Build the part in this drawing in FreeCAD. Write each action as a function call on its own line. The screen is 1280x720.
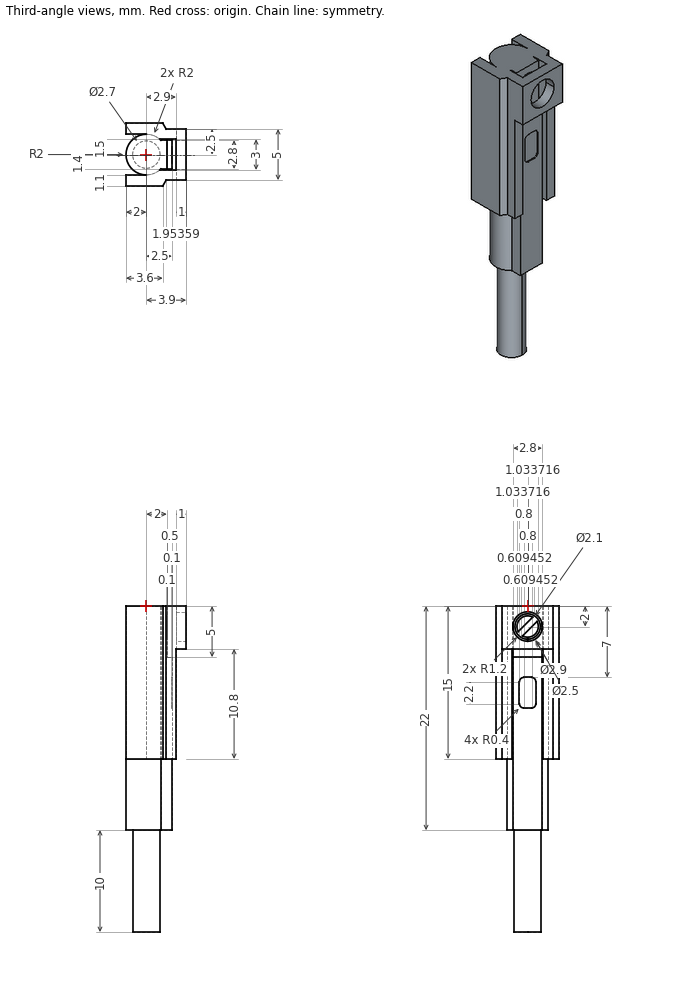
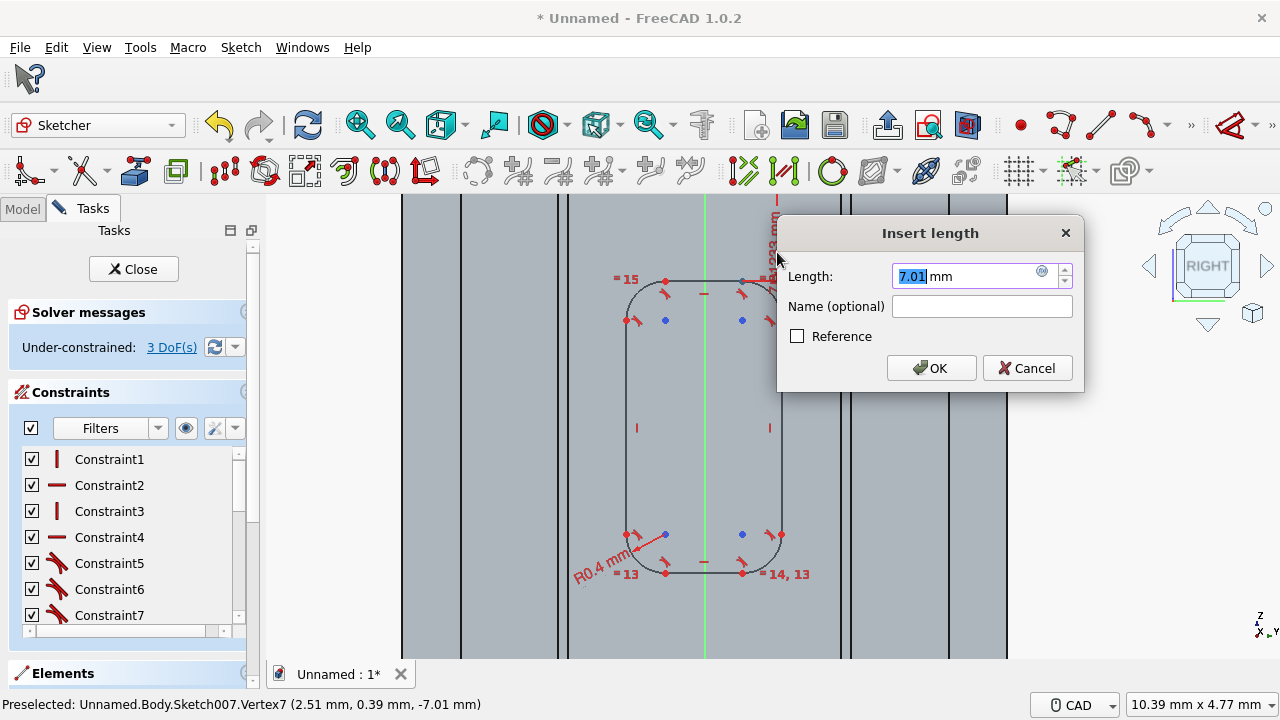
text(7)
key(Return)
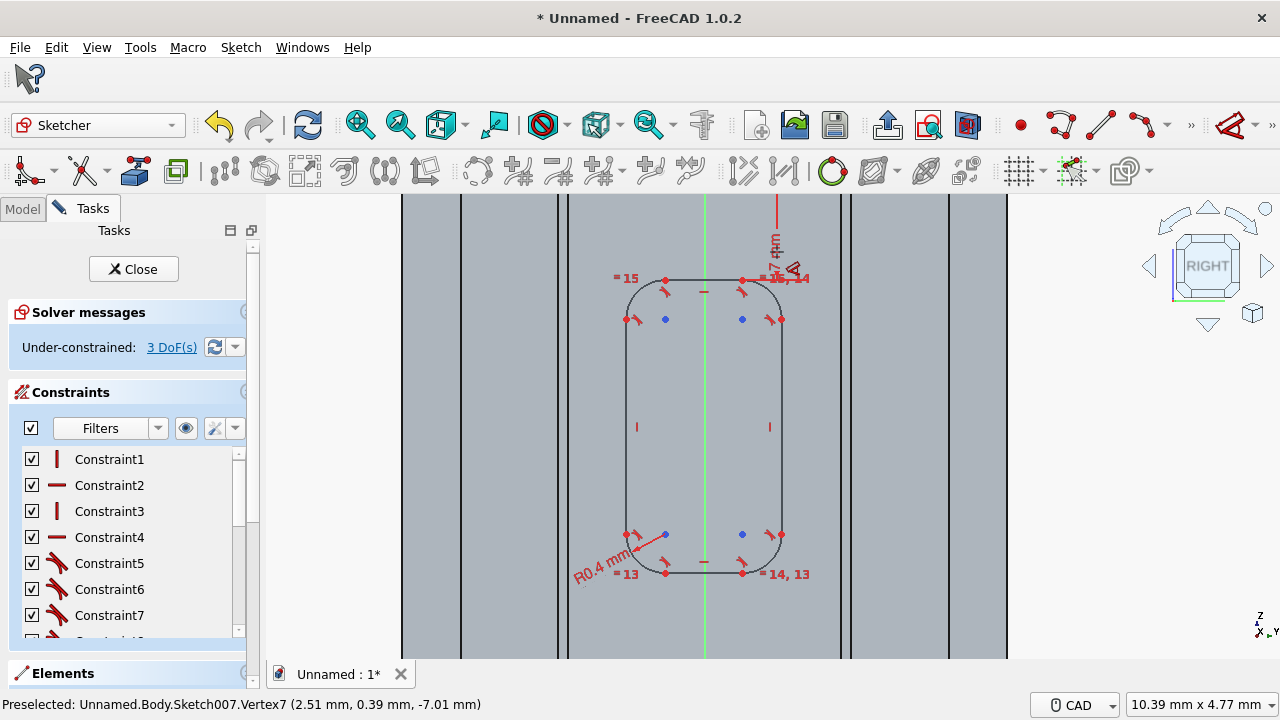
click(626, 384)
click(592, 427)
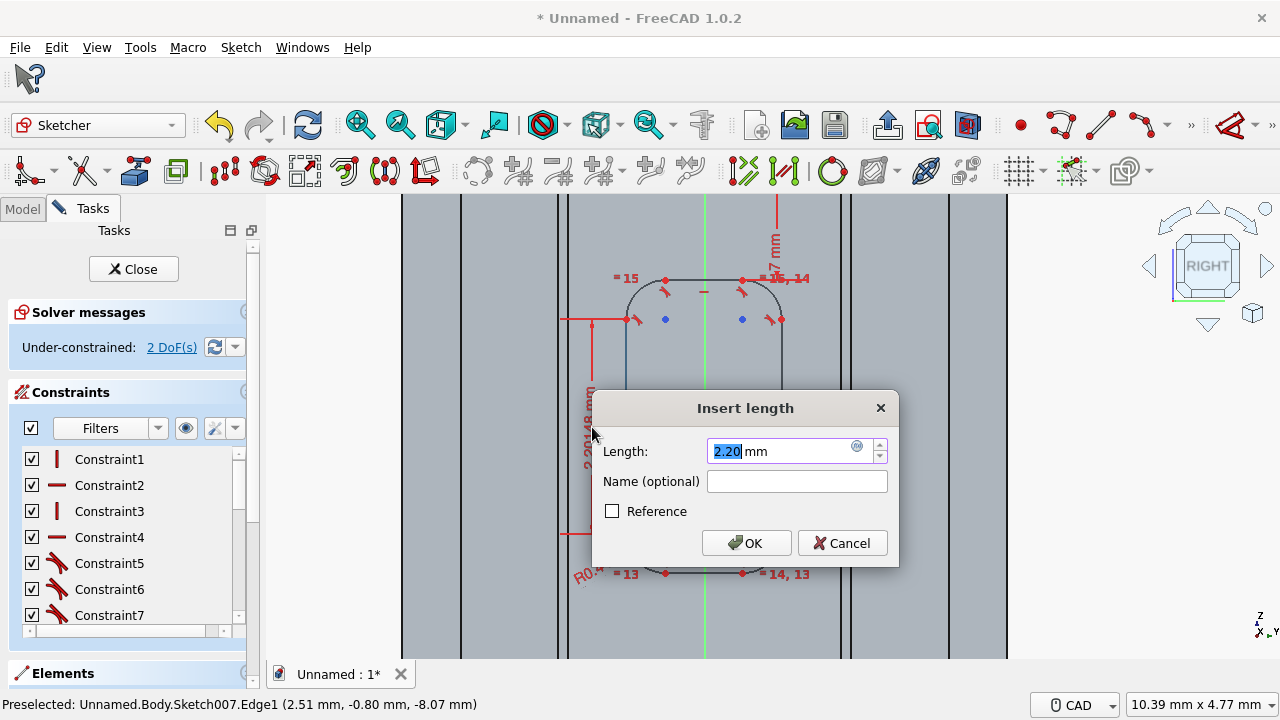
text(2.2)
key(Return)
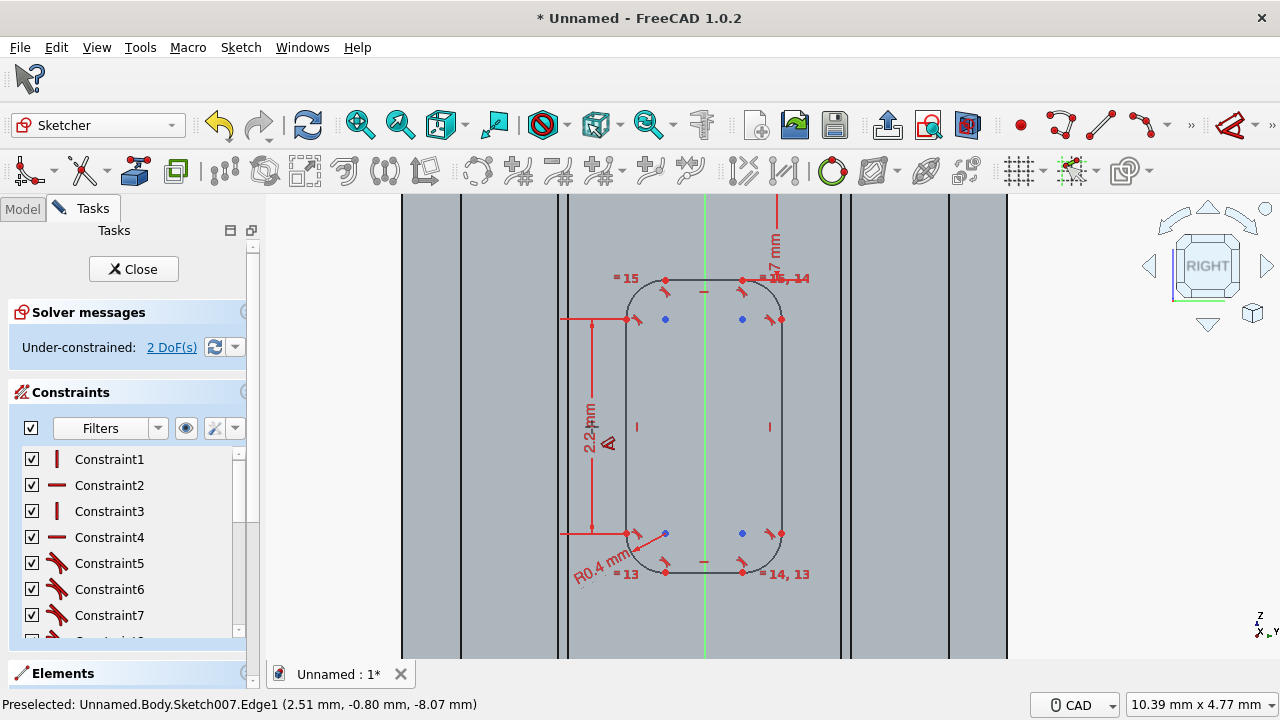
click(689, 573)
click(686, 607)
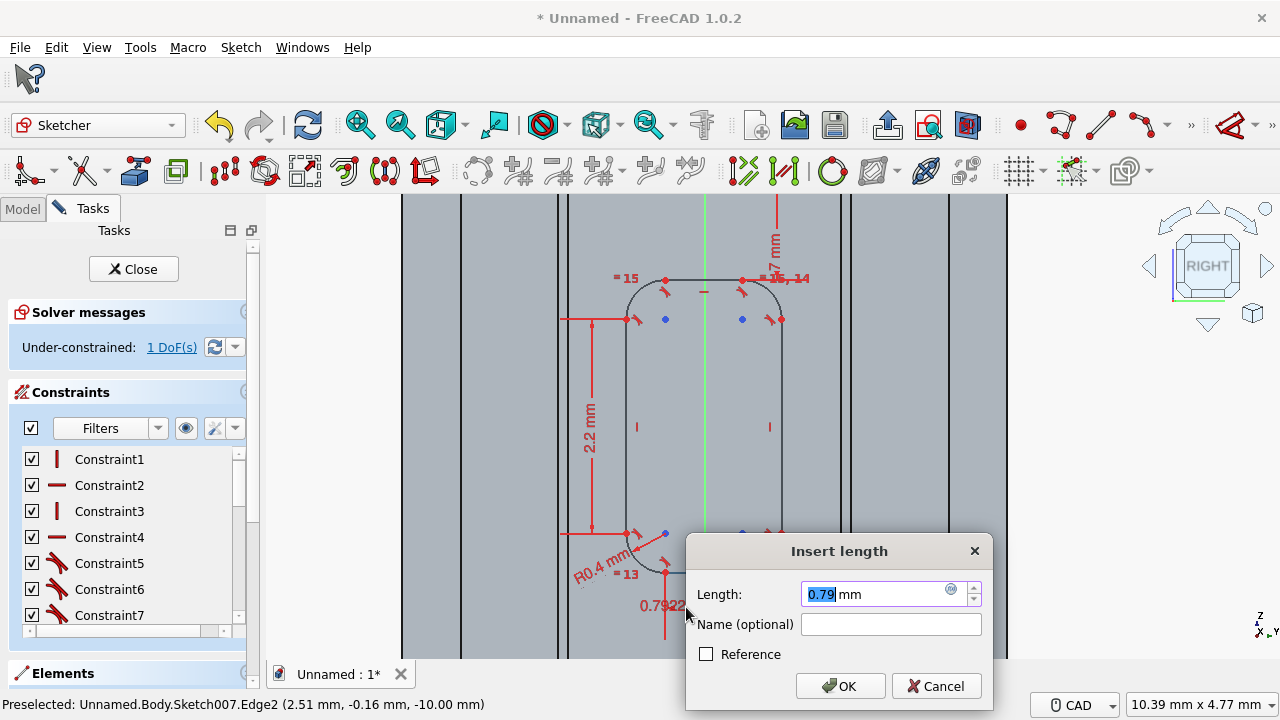
text(0.8)
key(Return)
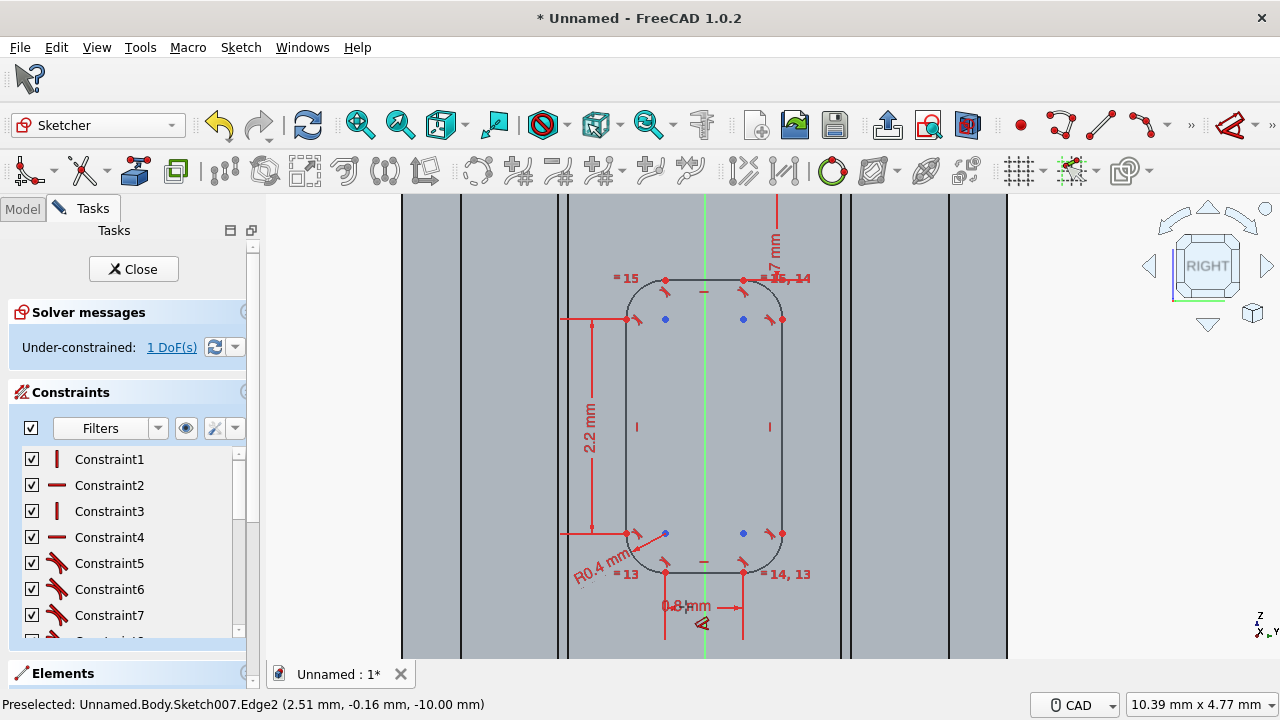
click(626, 319)
click(666, 353)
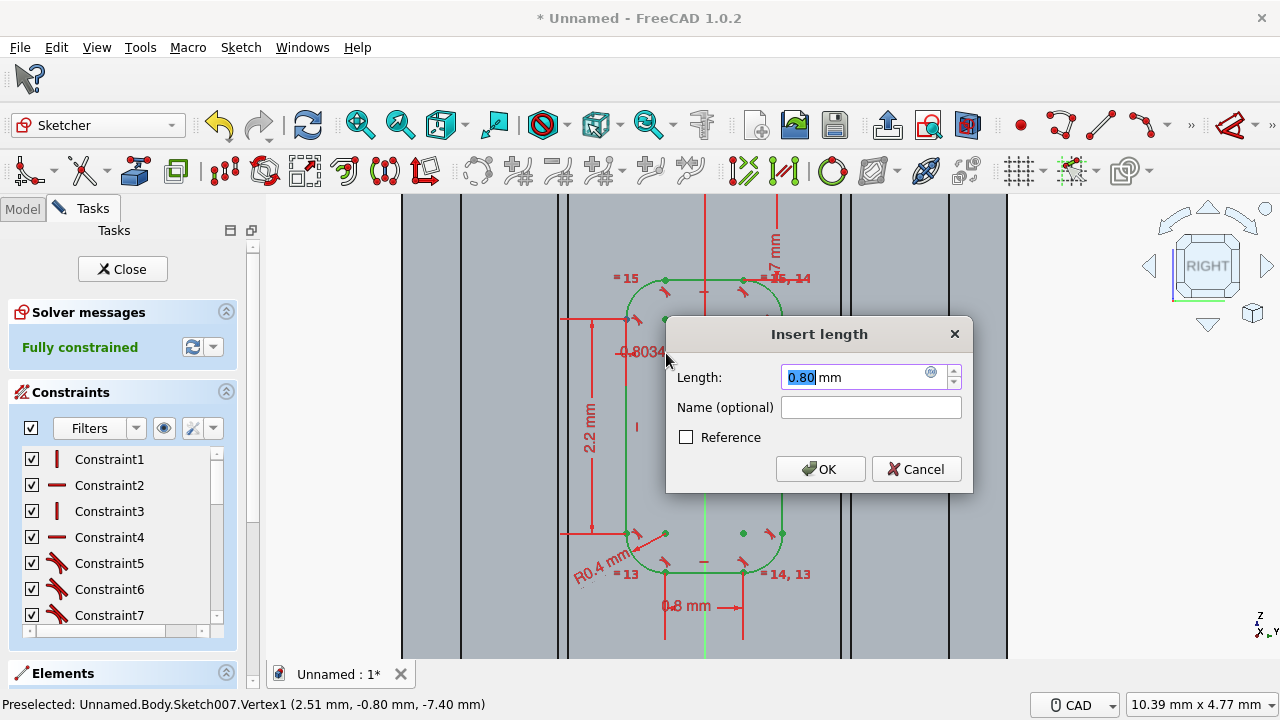
text(0.8)
key(Return)
key(Escape)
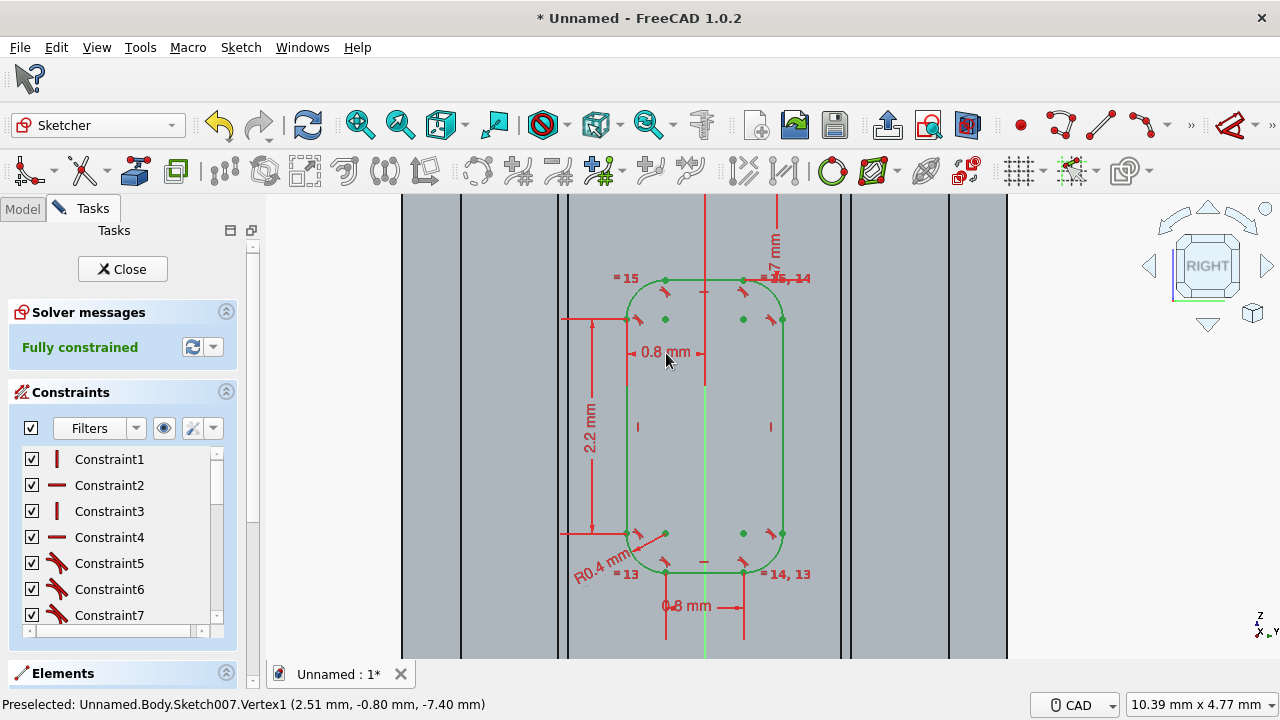
click(123, 269)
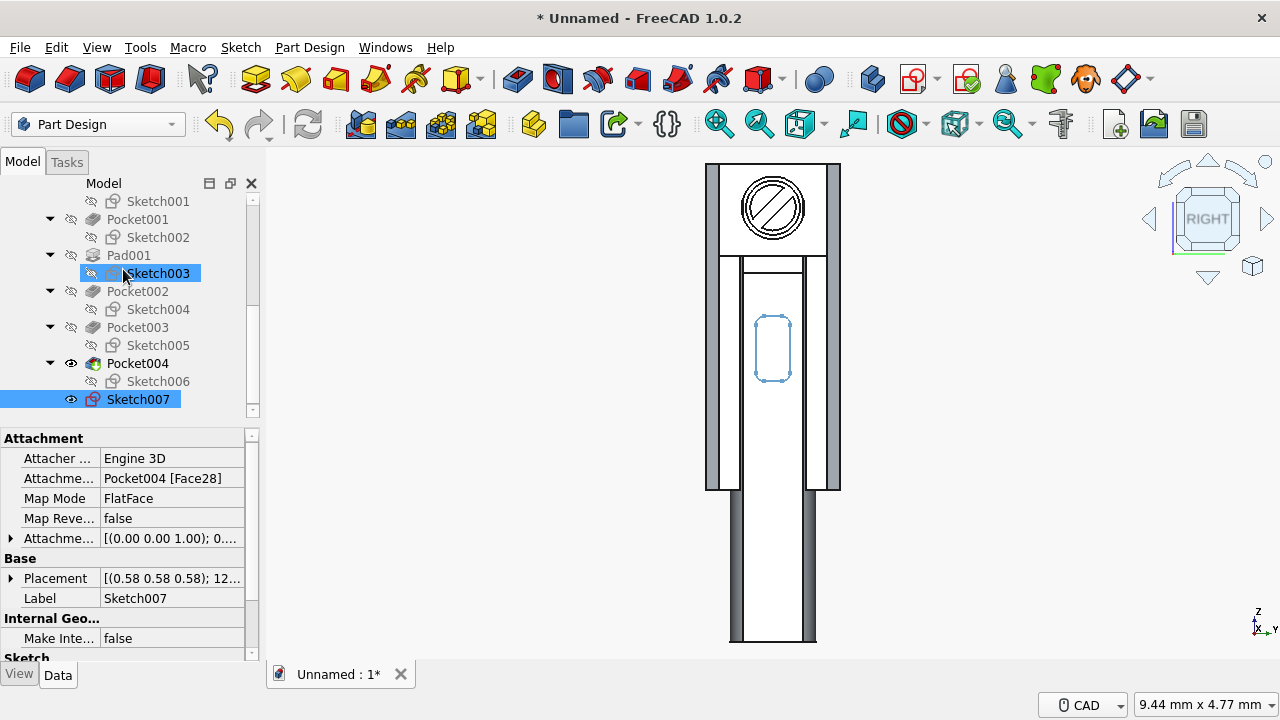
click(518, 80)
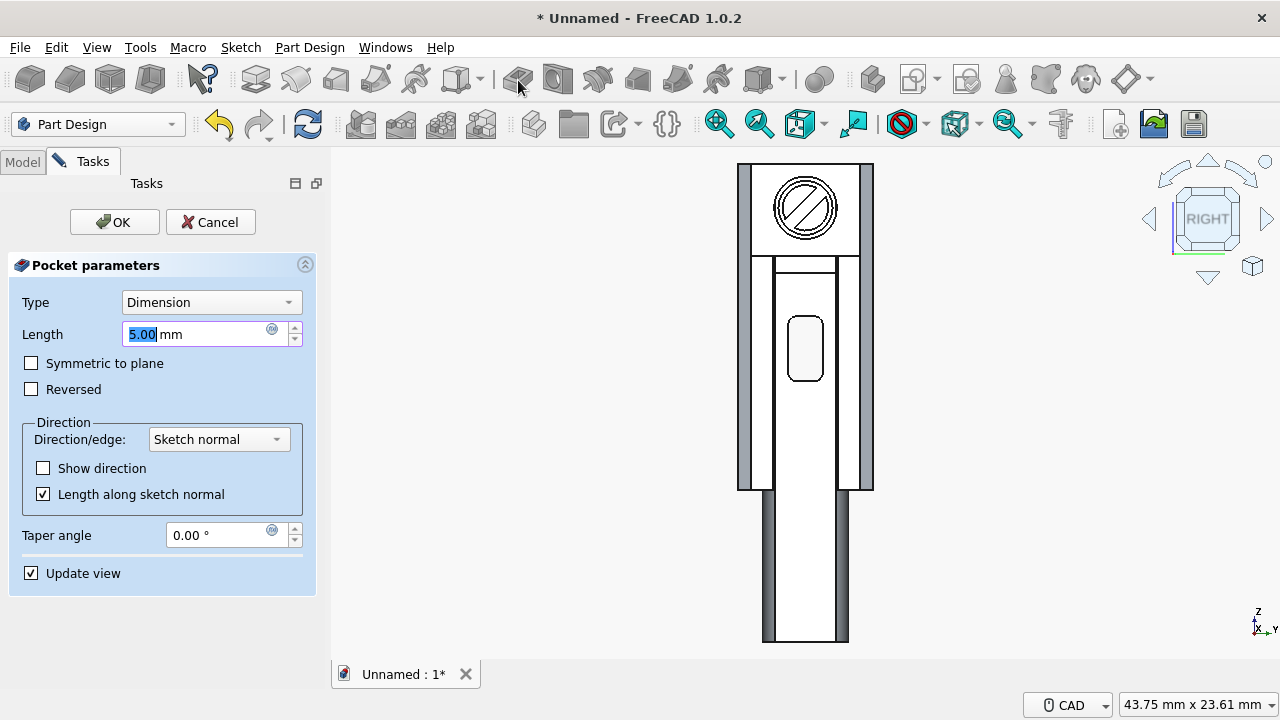
text(0.1)
key(Tab)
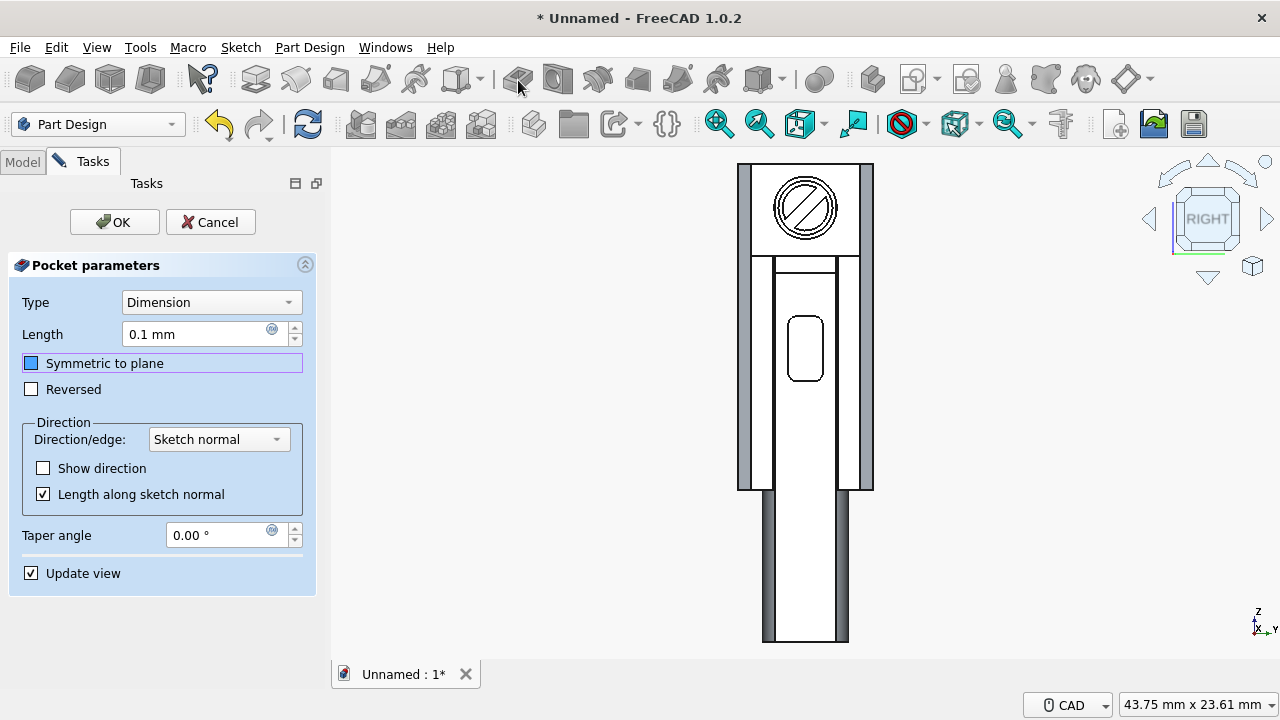
click(115, 222)